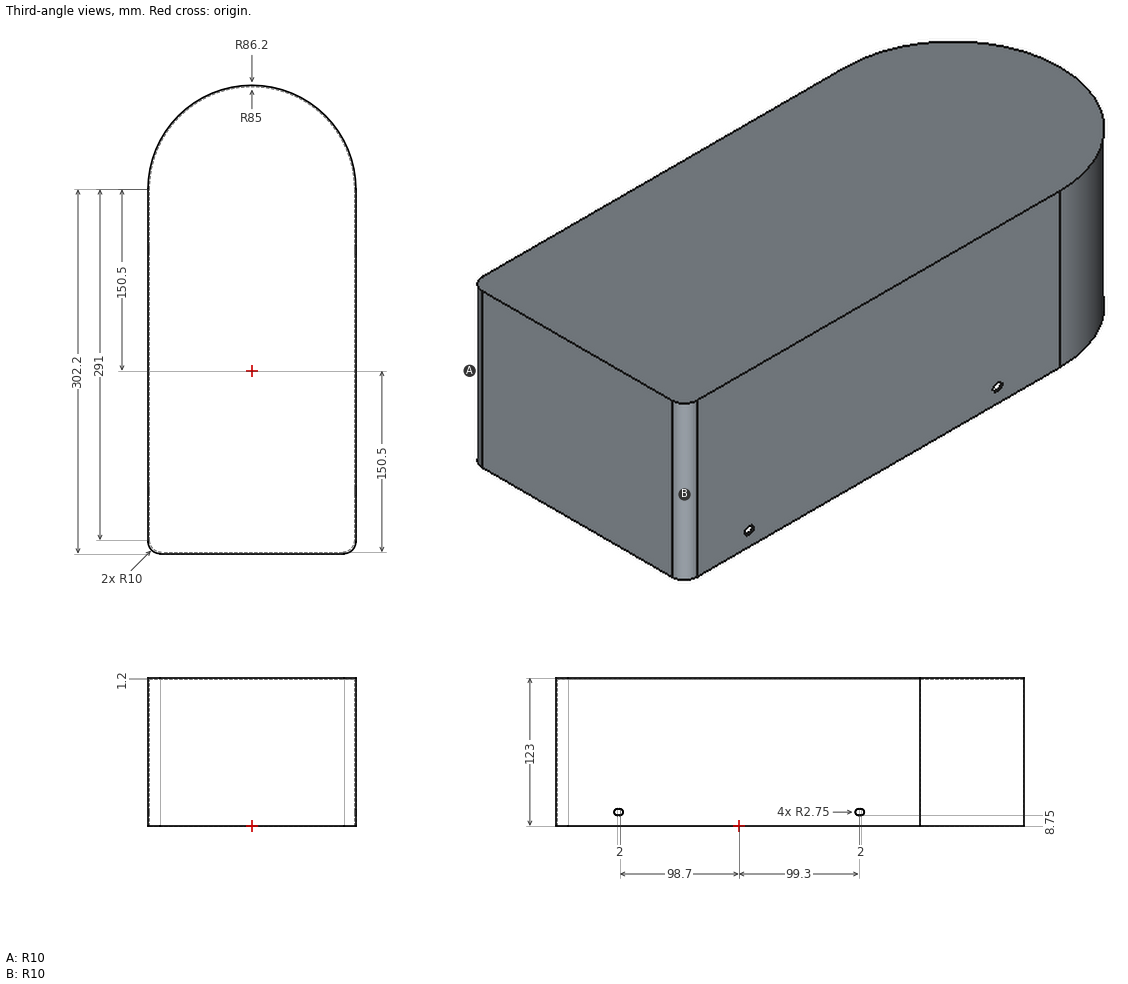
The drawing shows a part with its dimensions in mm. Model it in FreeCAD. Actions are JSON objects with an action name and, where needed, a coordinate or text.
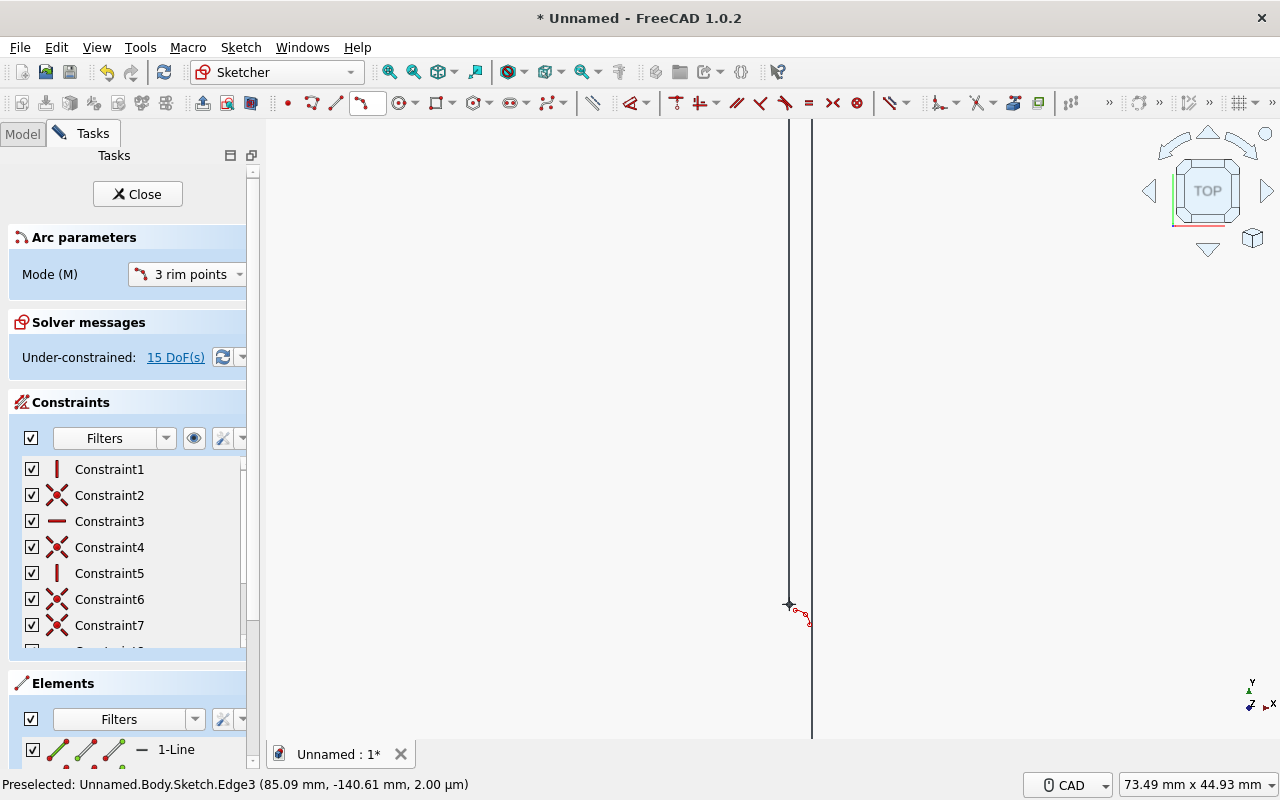
{"action": "scroll", "coordinate": [792, 618], "scroll_direction": "down", "scroll_amount": 13}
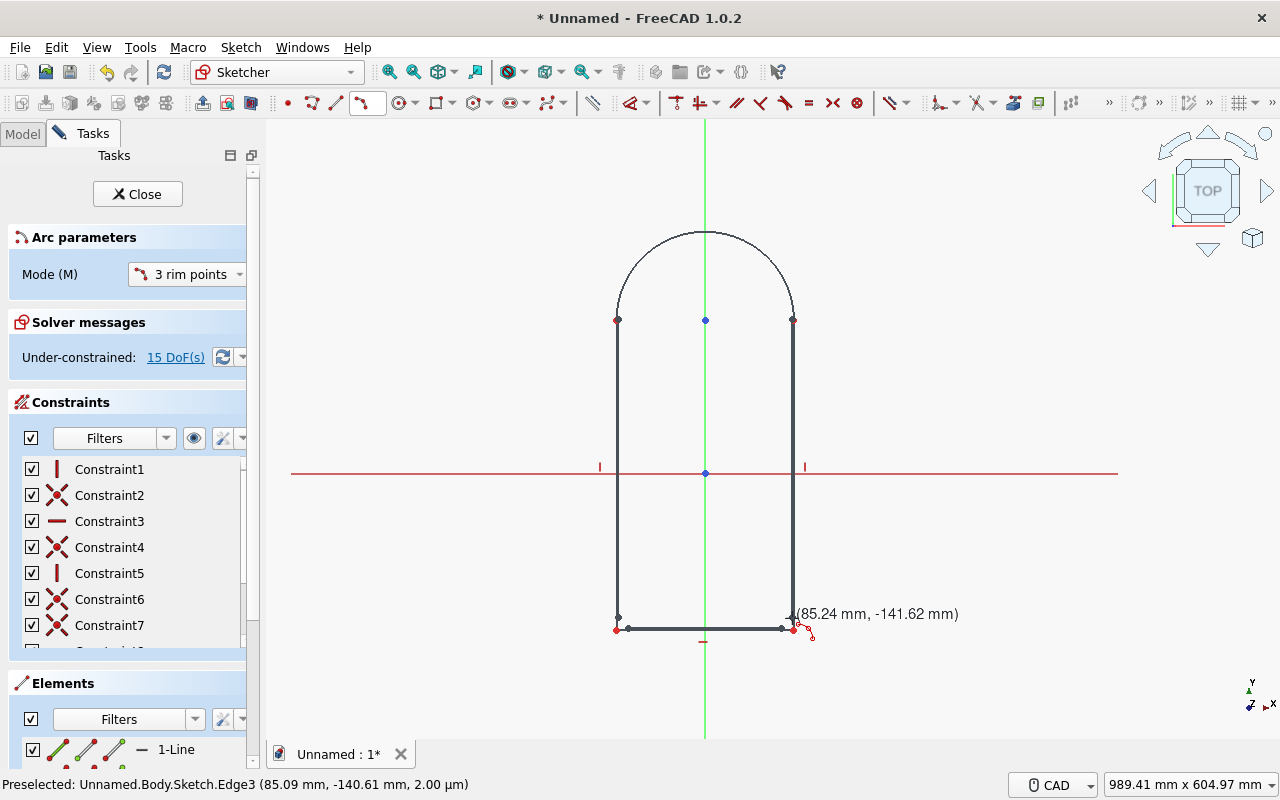
{"action": "scroll", "coordinate": [628, 628], "scroll_direction": "up", "scroll_amount": 13}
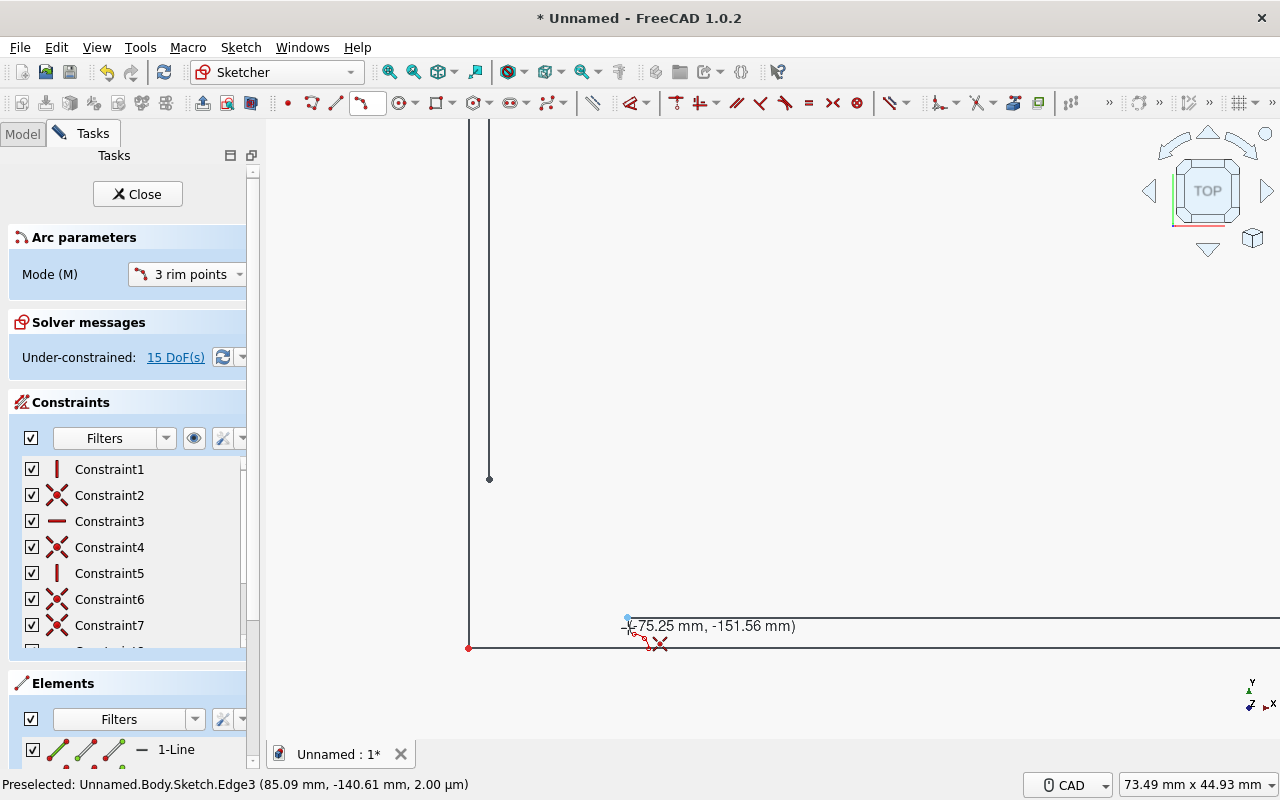
{"action": "left_click", "coordinate": [627, 618]}
{"action": "left_click", "coordinate": [489, 480]}
{"action": "left_click", "coordinate": [529, 576]}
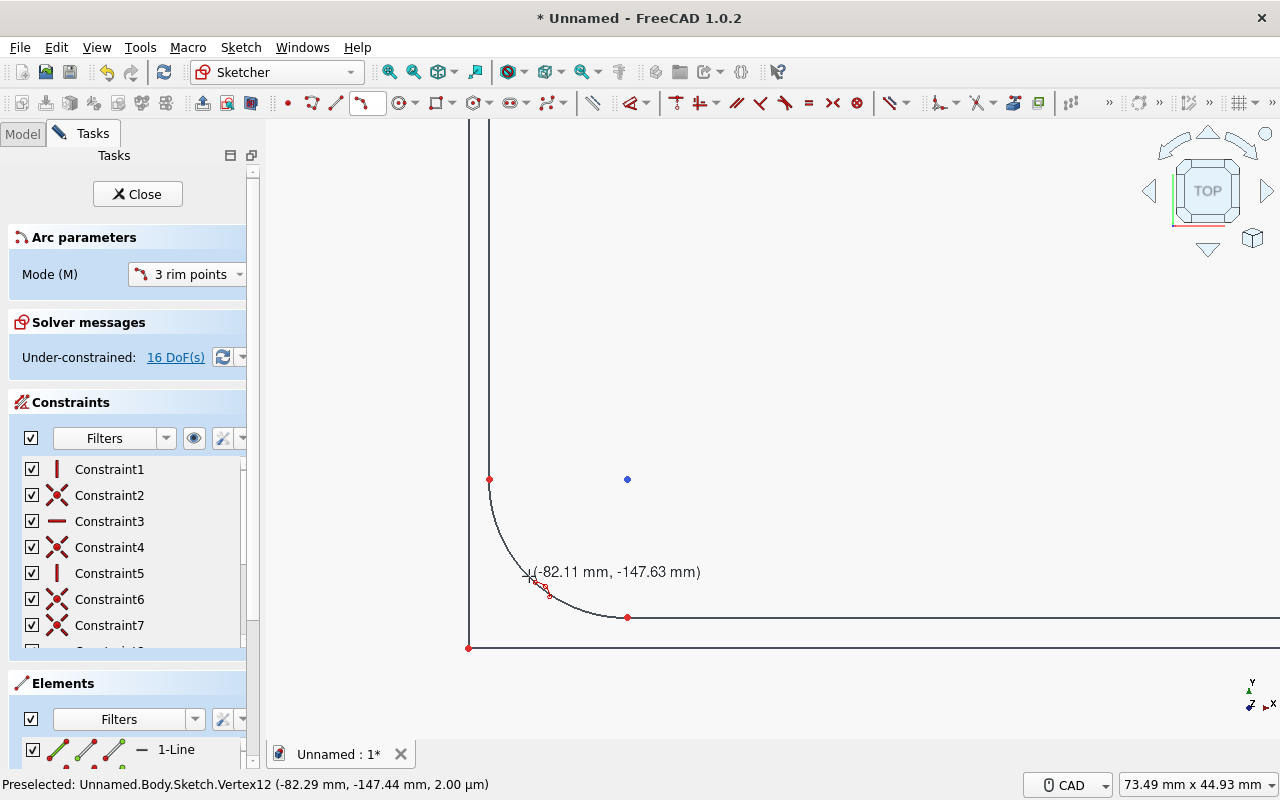
{"action": "scroll", "coordinate": [628, 628], "scroll_direction": "down", "scroll_amount": 13}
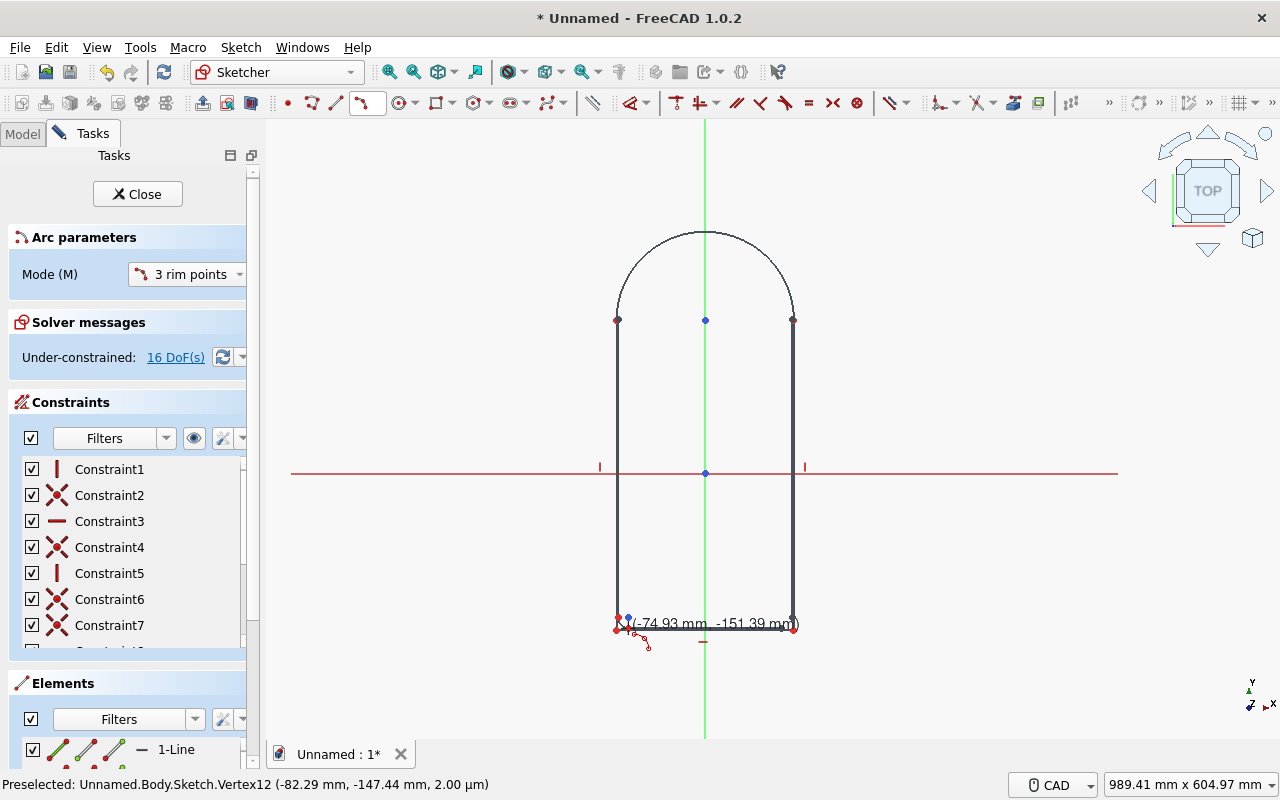
{"action": "scroll", "coordinate": [618, 319], "scroll_direction": "up", "scroll_amount": 13}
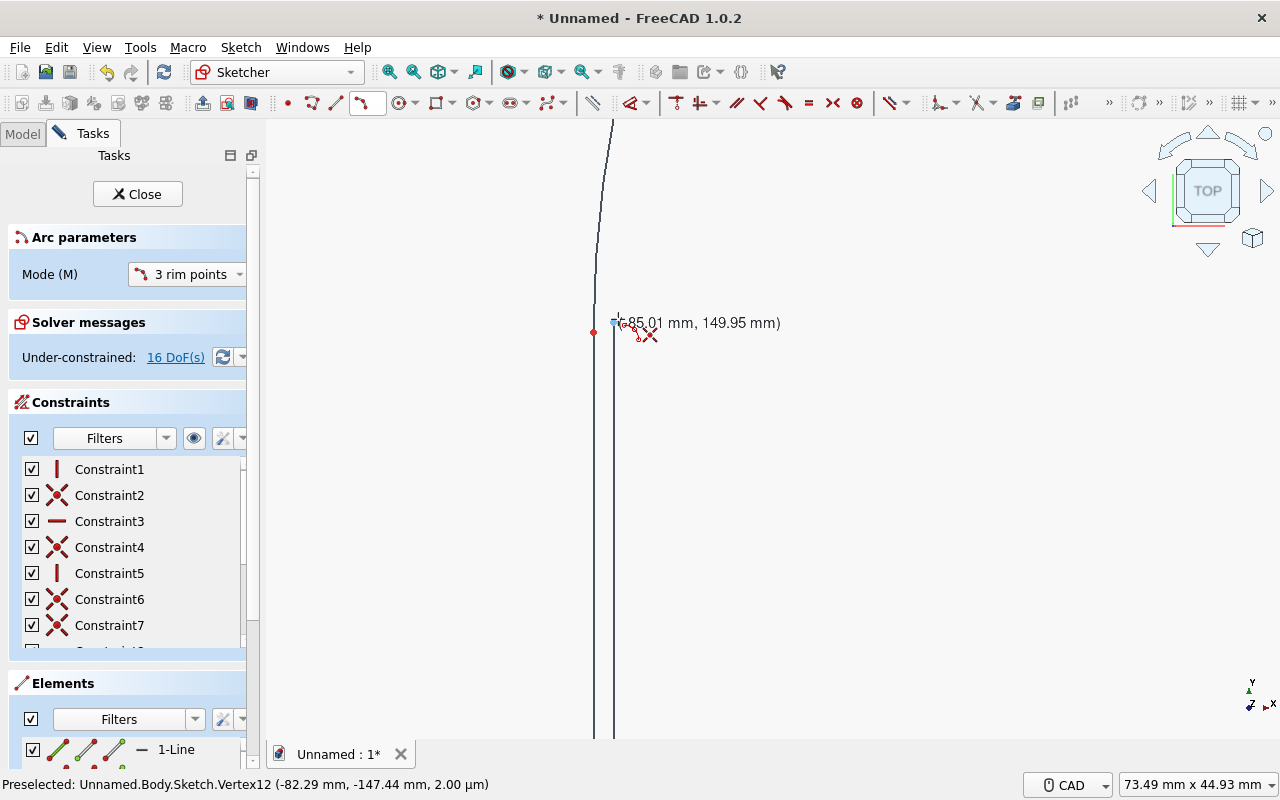
{"action": "left_click", "coordinate": [614, 322]}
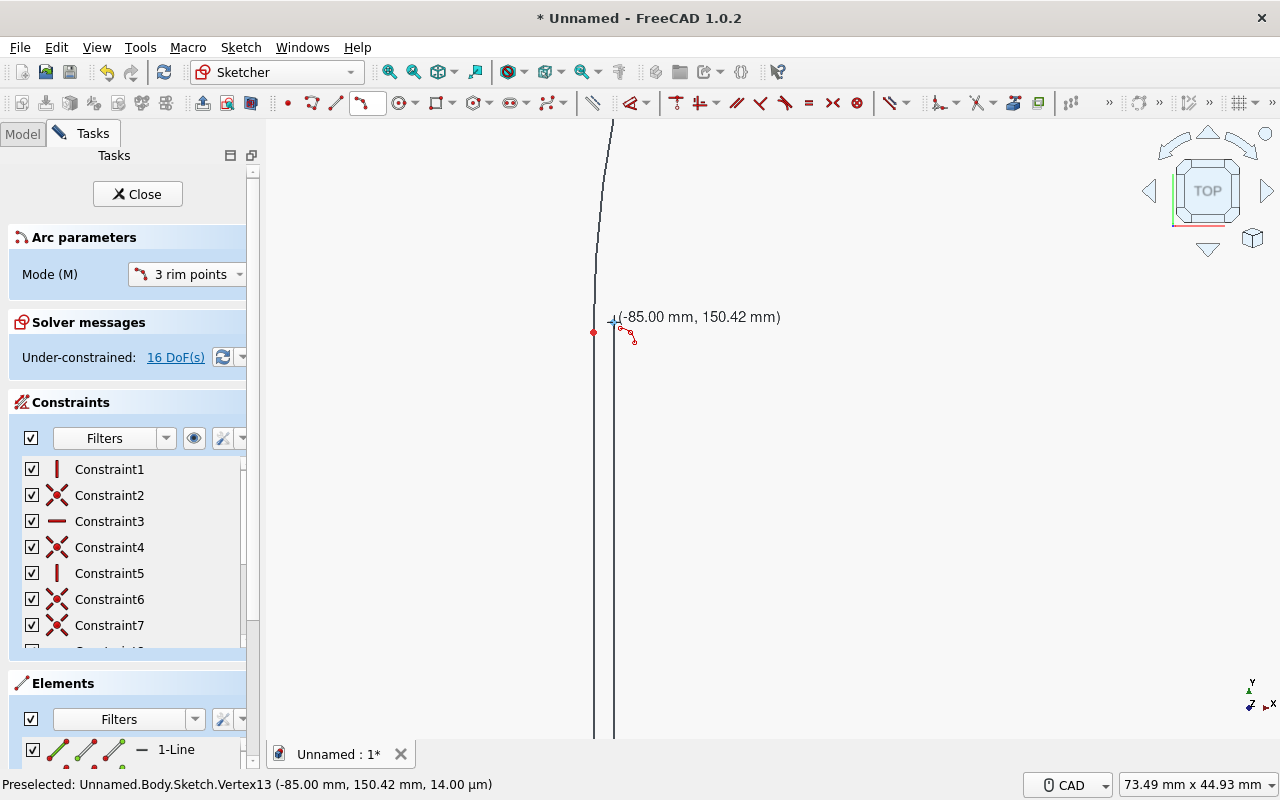
{"action": "scroll", "coordinate": [618, 318], "scroll_direction": "down", "scroll_amount": 13}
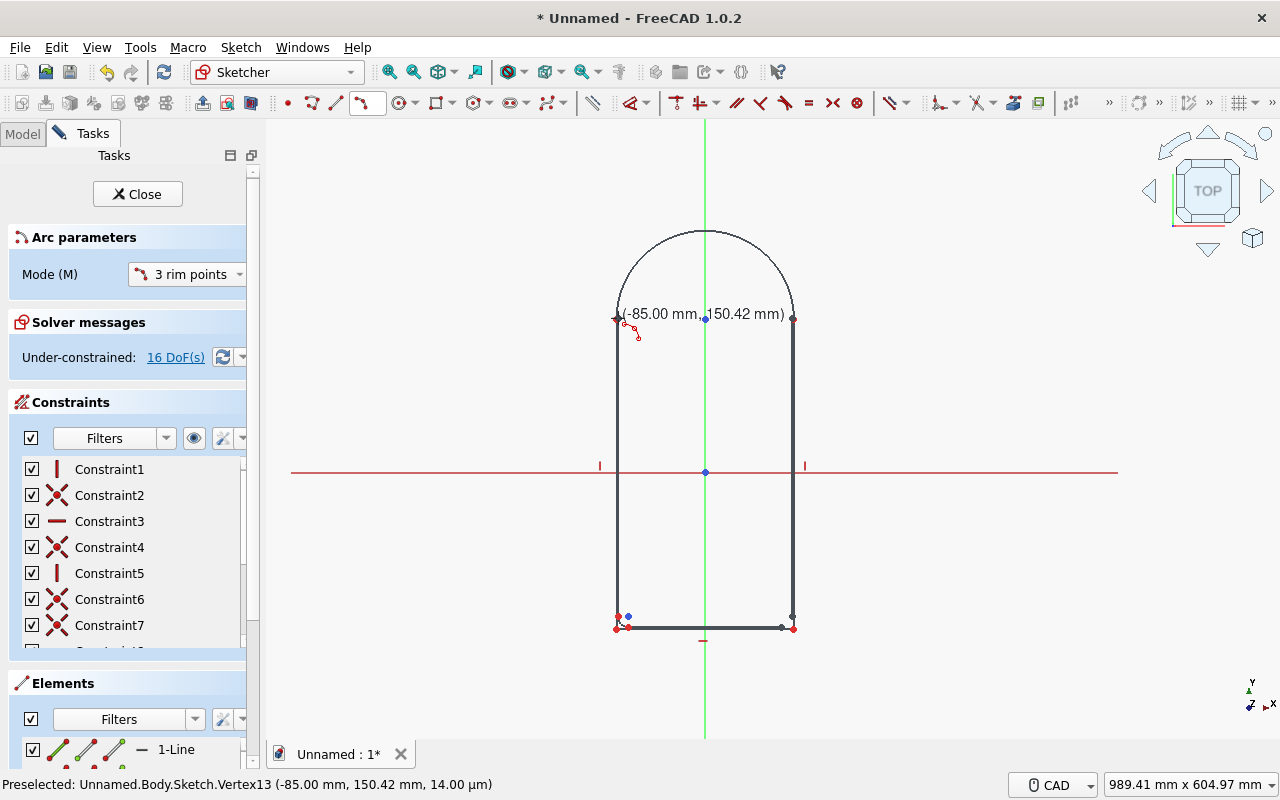
{"action": "scroll", "coordinate": [792, 319], "scroll_direction": "up", "scroll_amount": 13}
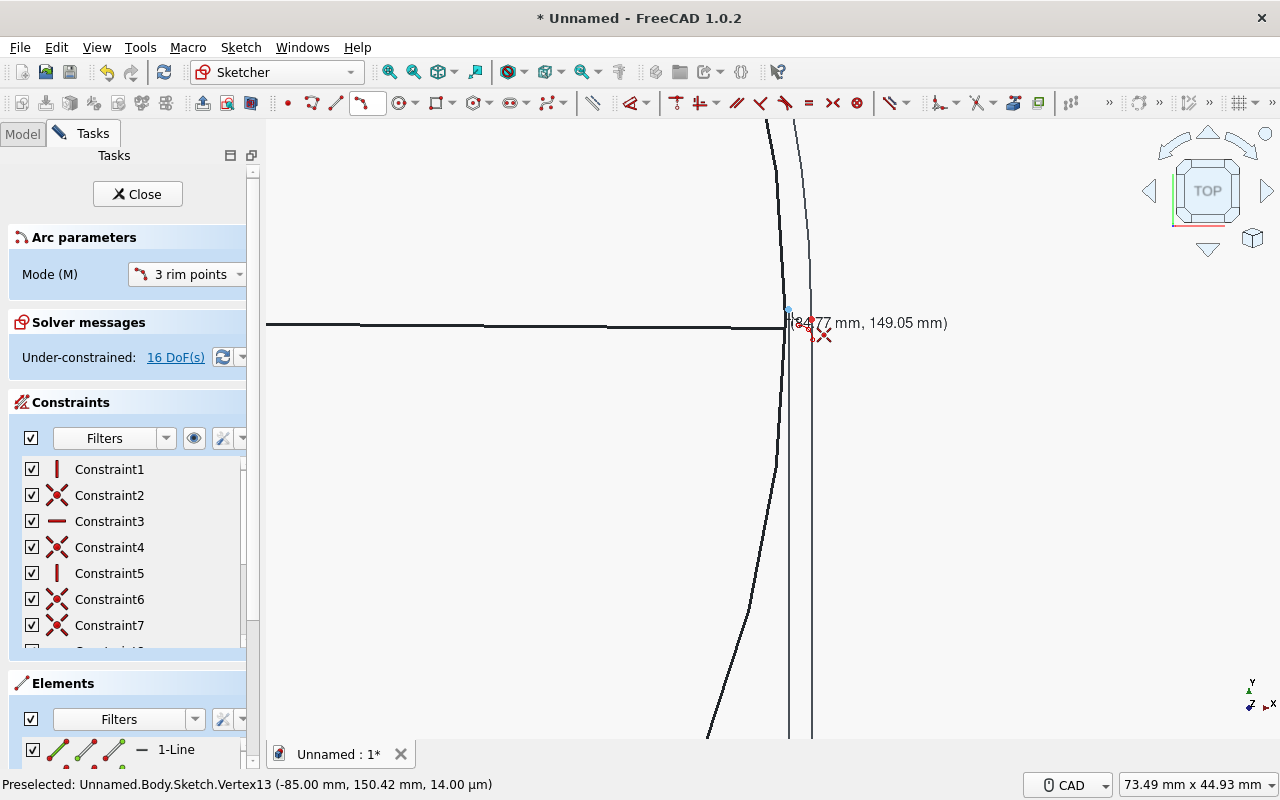
{"action": "left_click", "coordinate": [789, 309]}